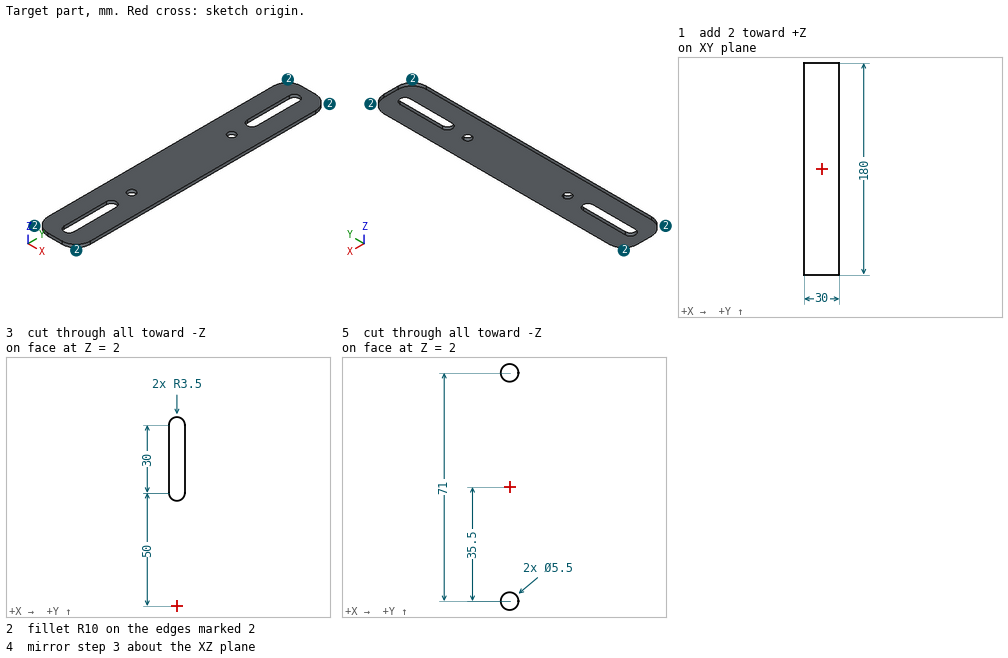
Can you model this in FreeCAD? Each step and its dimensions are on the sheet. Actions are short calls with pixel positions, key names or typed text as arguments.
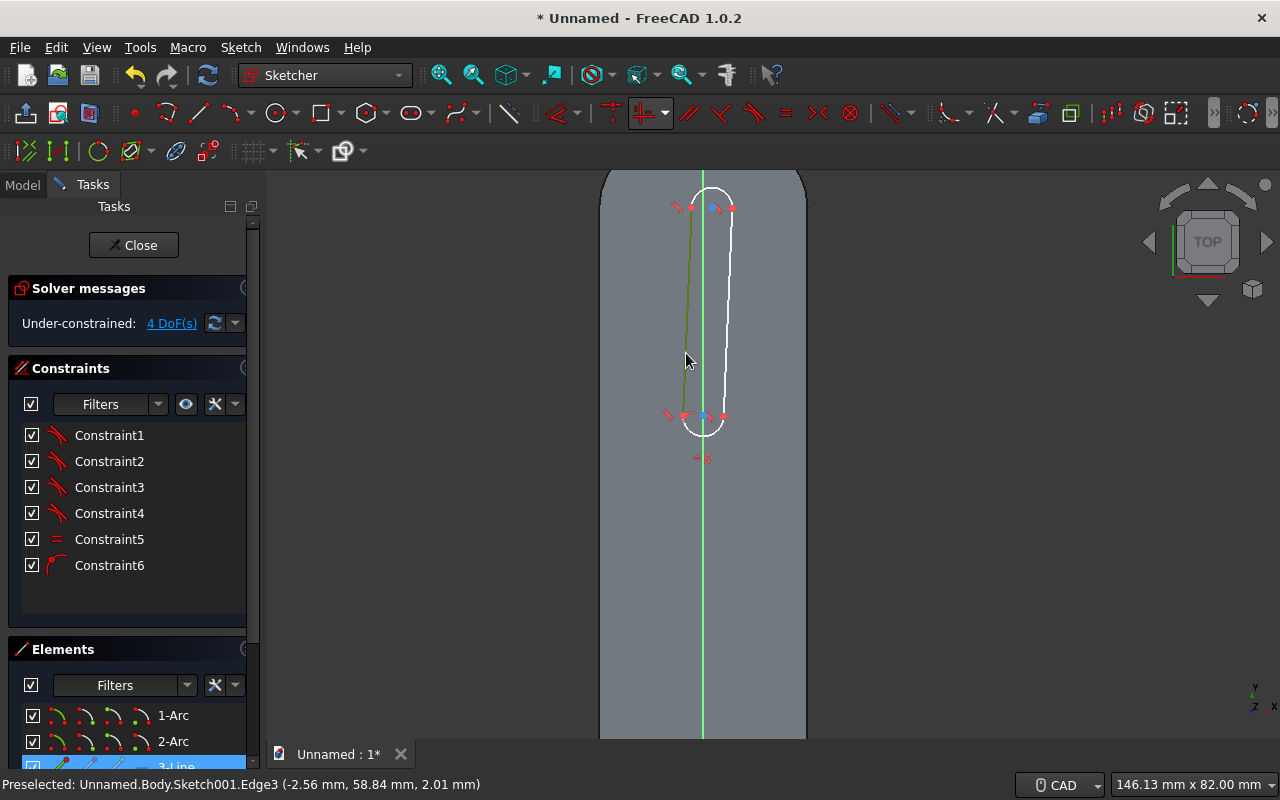
key(v)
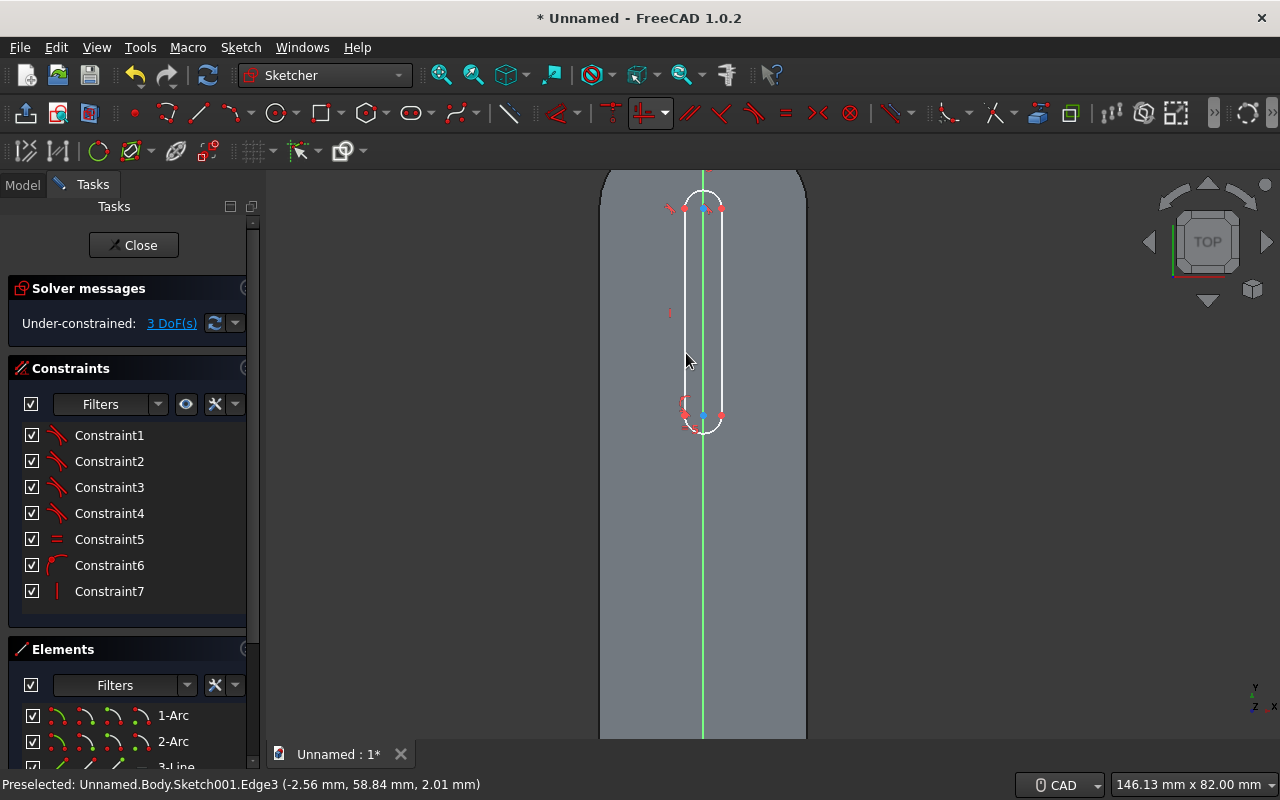
click(556, 114)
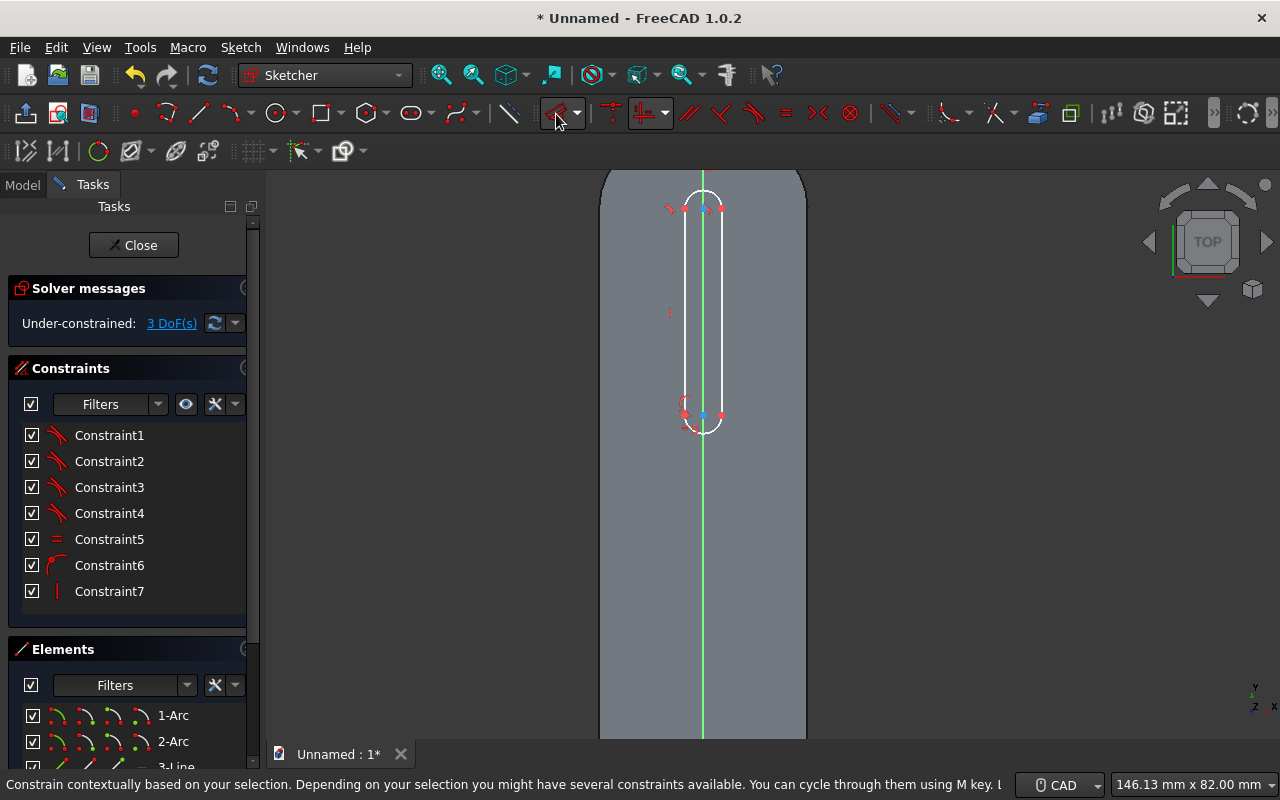
scroll(693, 430, up, 3)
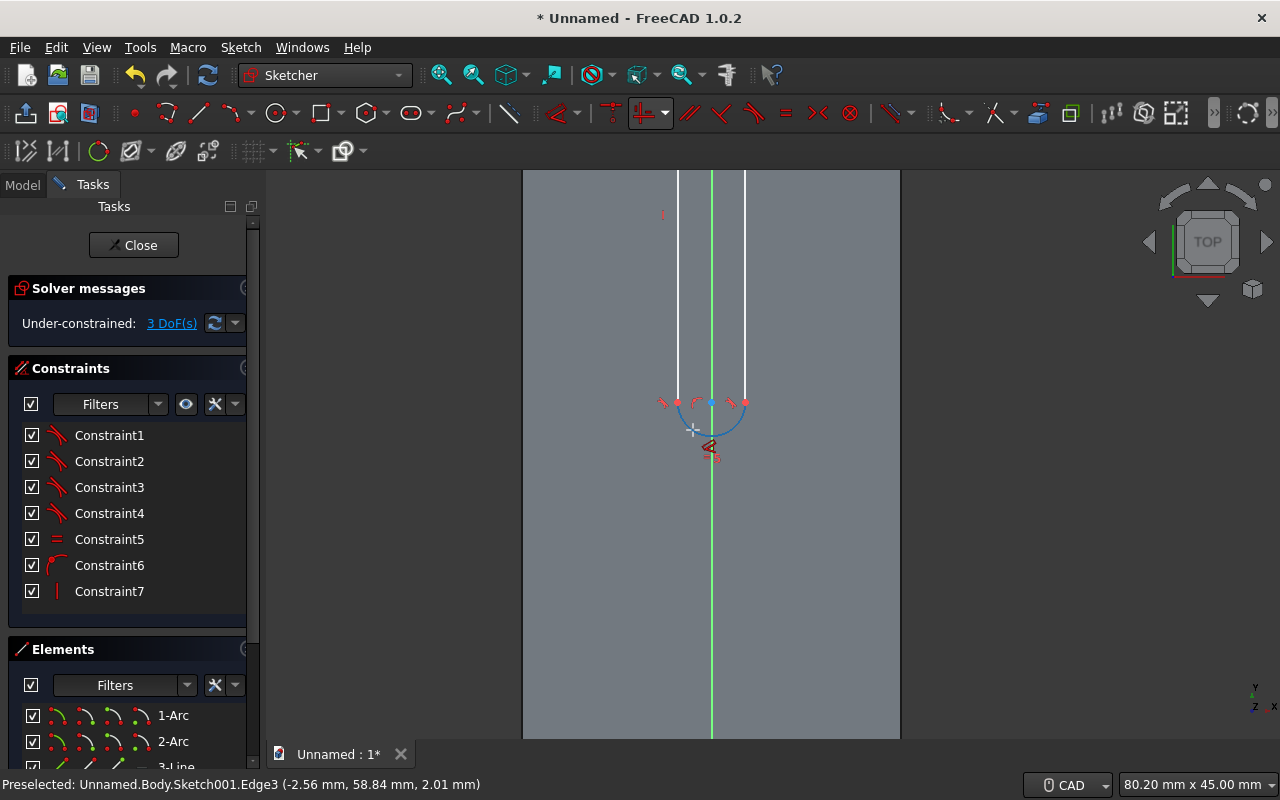
click(692, 430)
click(673, 456)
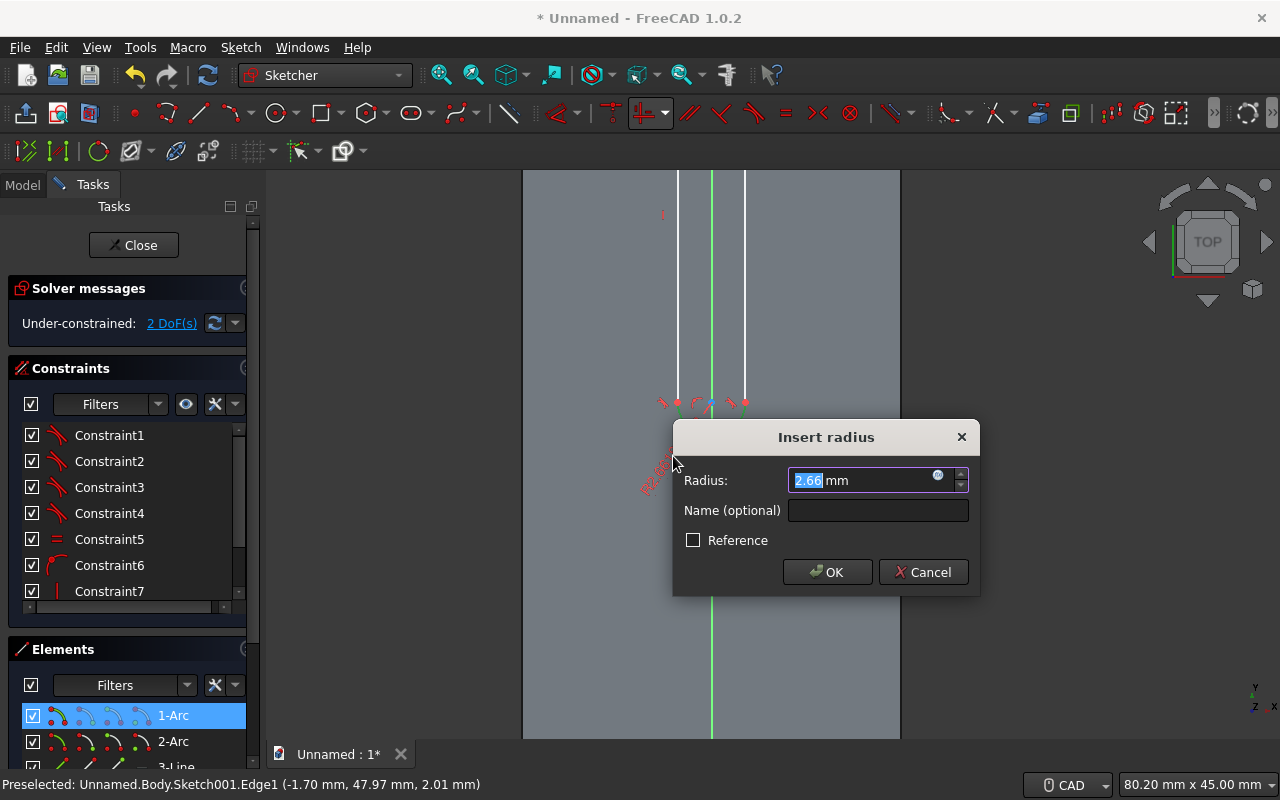
text(3.5)
key(Return)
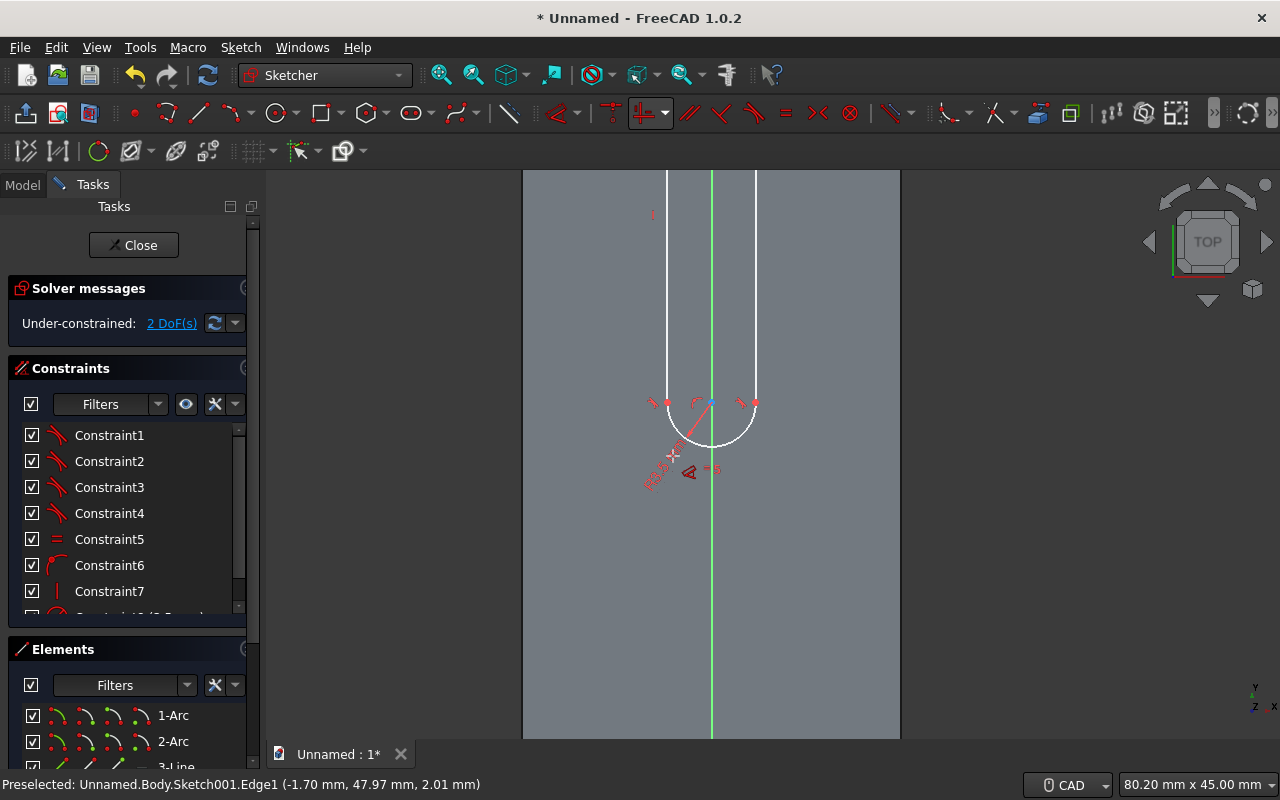
click(667, 290)
click(633, 300)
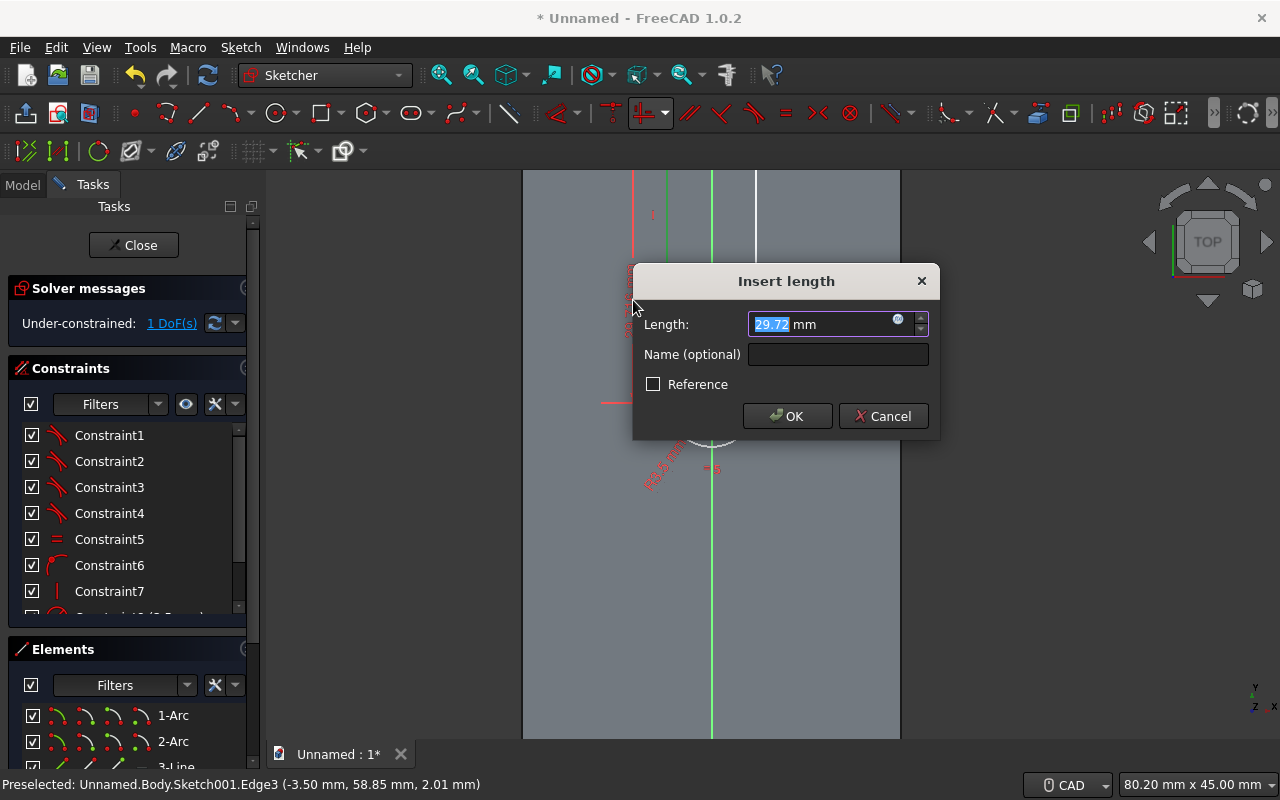
text(30)
key(Return)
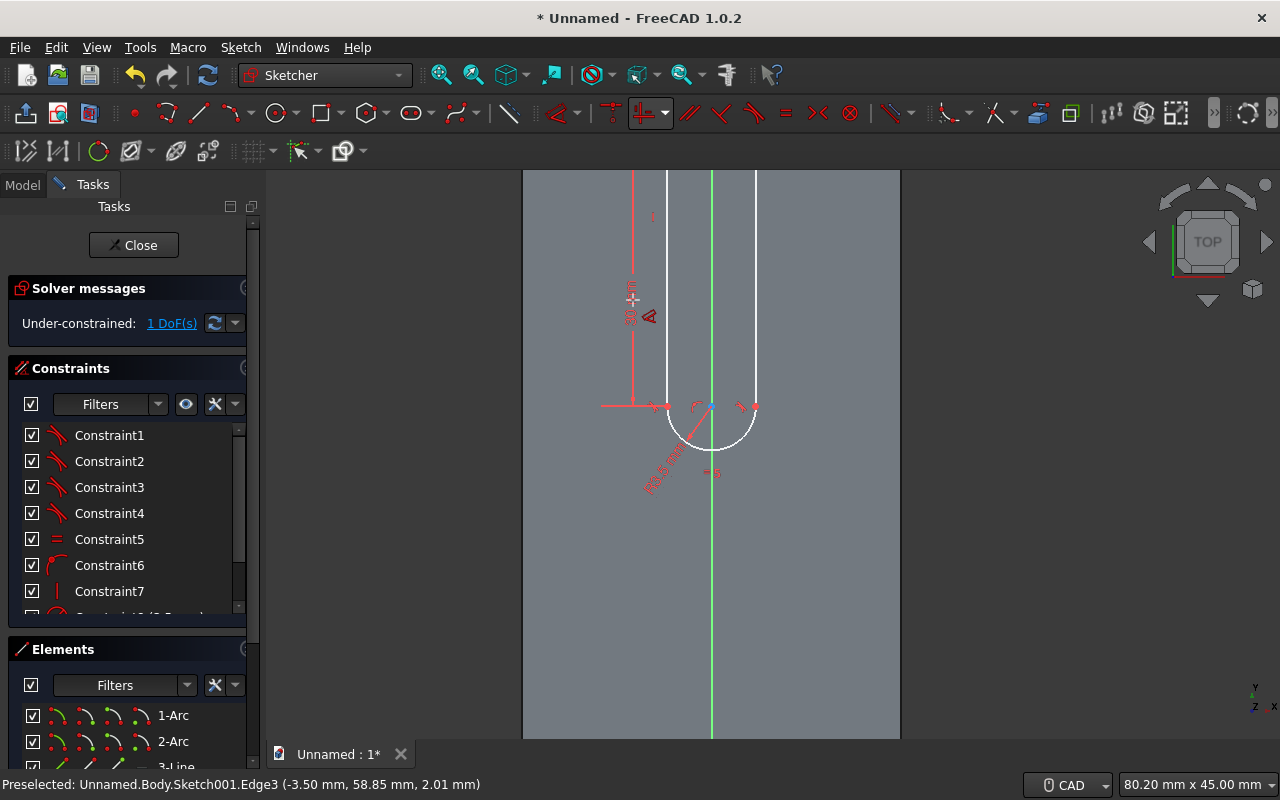
click(667, 406)
click(633, 559)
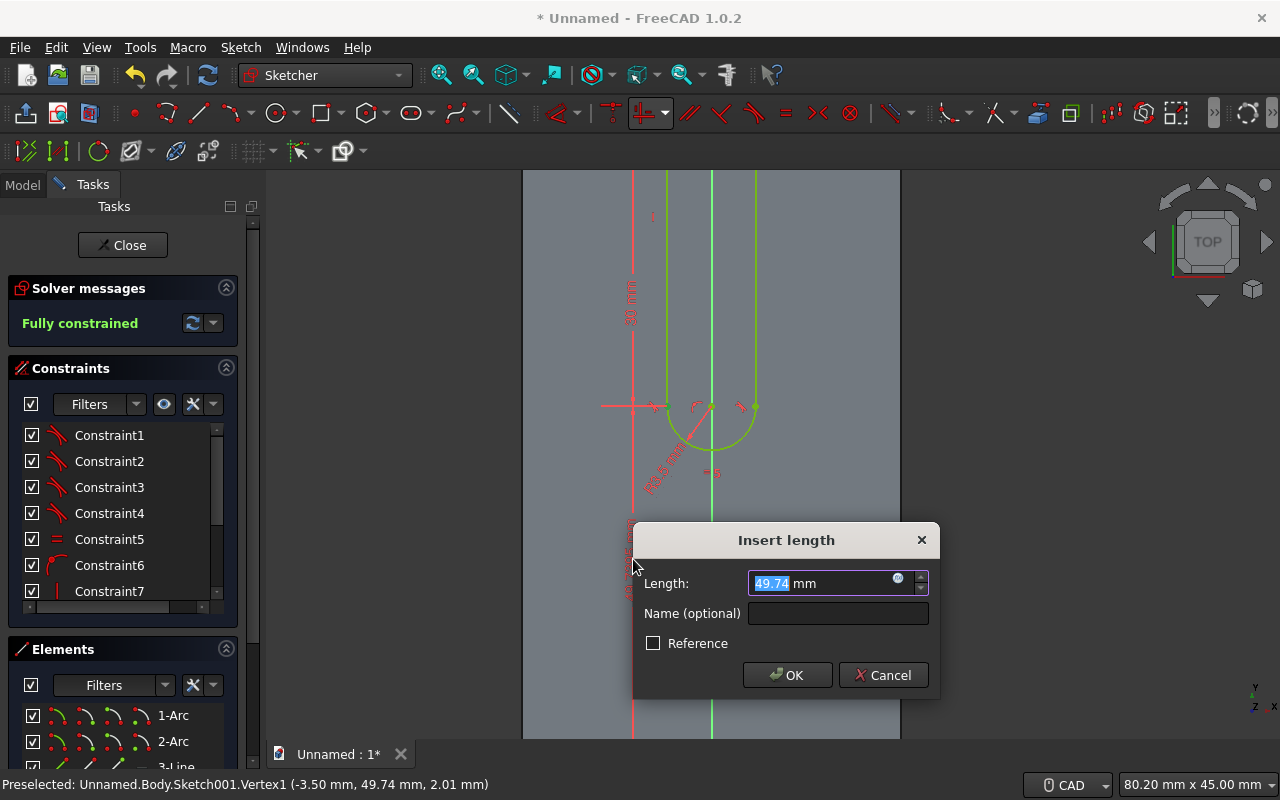
text(50)
key(Return)
key(Escape)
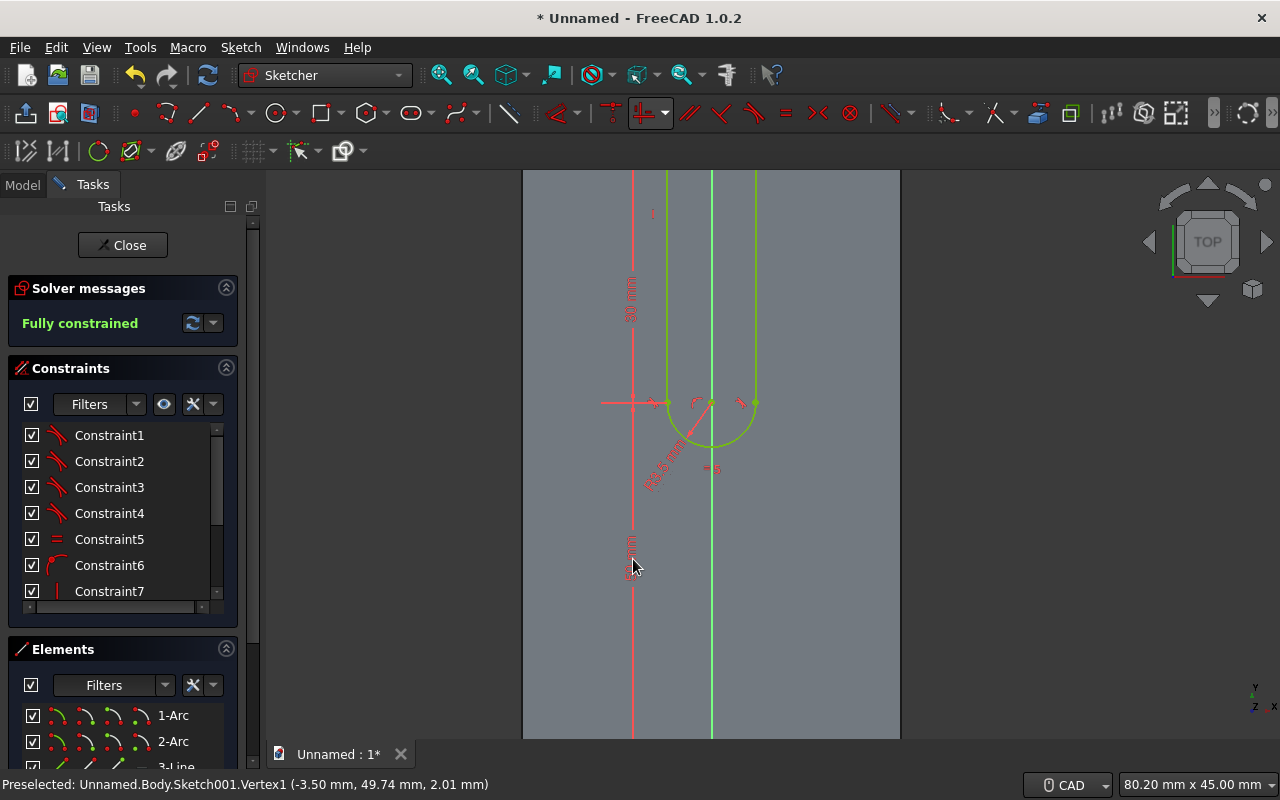
click(123, 245)